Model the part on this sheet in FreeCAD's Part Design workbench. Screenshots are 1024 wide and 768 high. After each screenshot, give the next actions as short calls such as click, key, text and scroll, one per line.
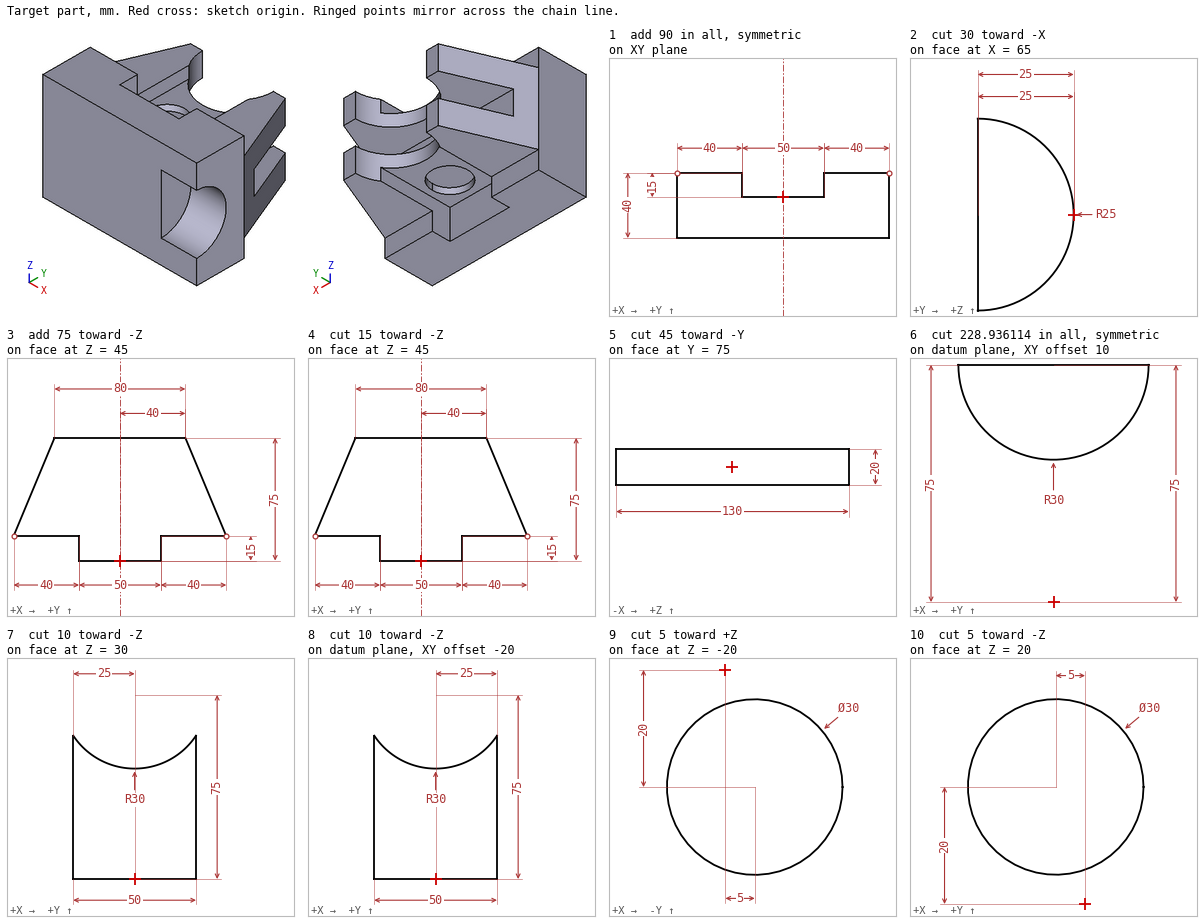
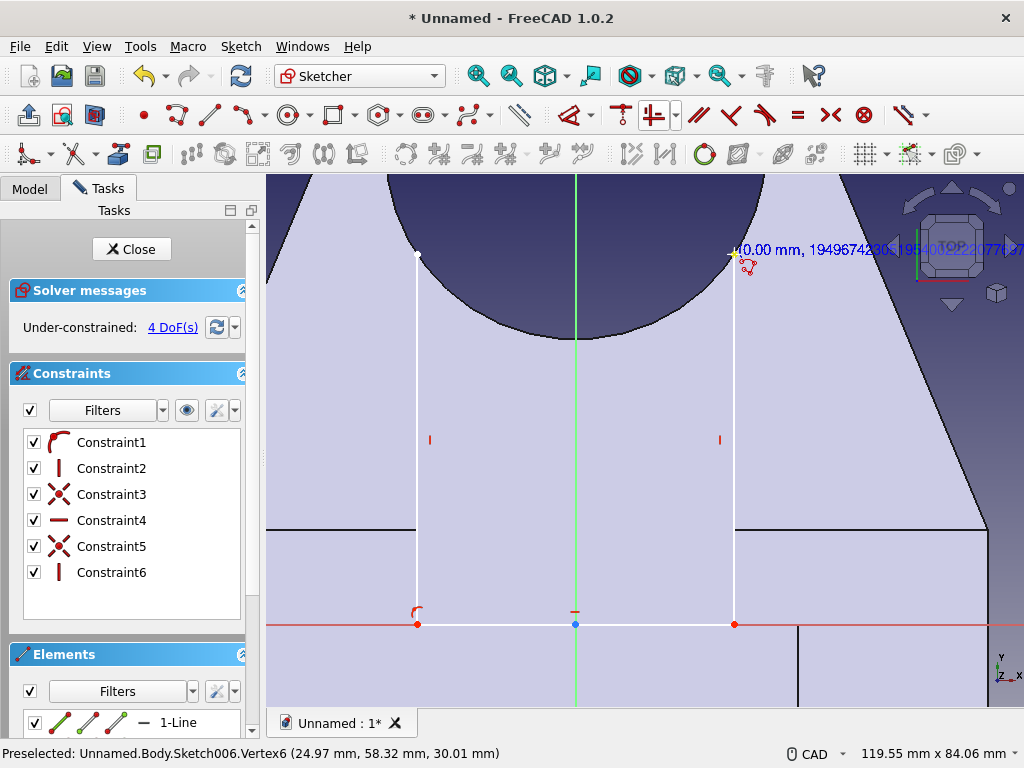
key(g)
key(3)
key(a)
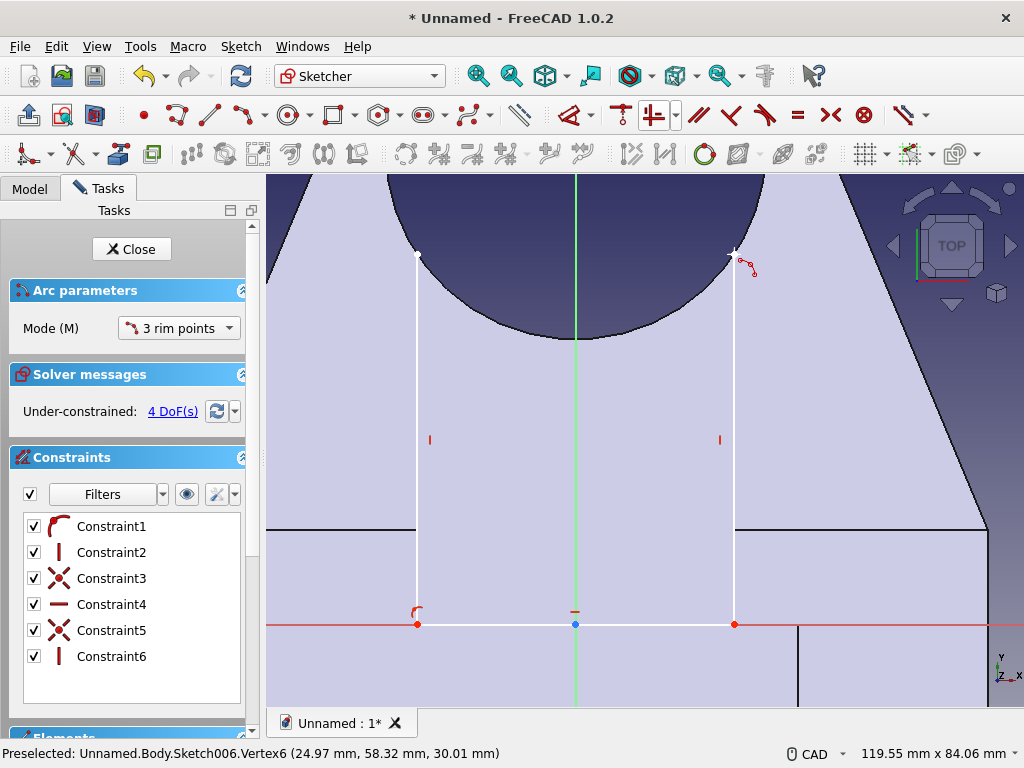
click(734, 255)
click(417, 255)
click(538, 336)
key(Escape)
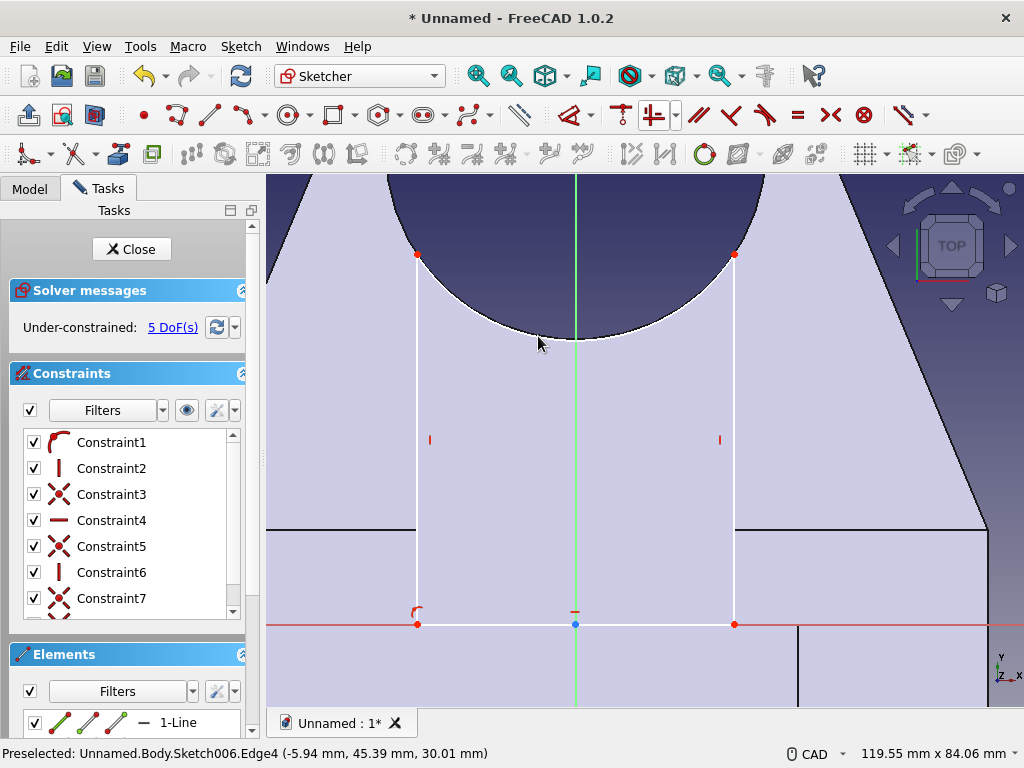
scroll(578, 547, down, 2)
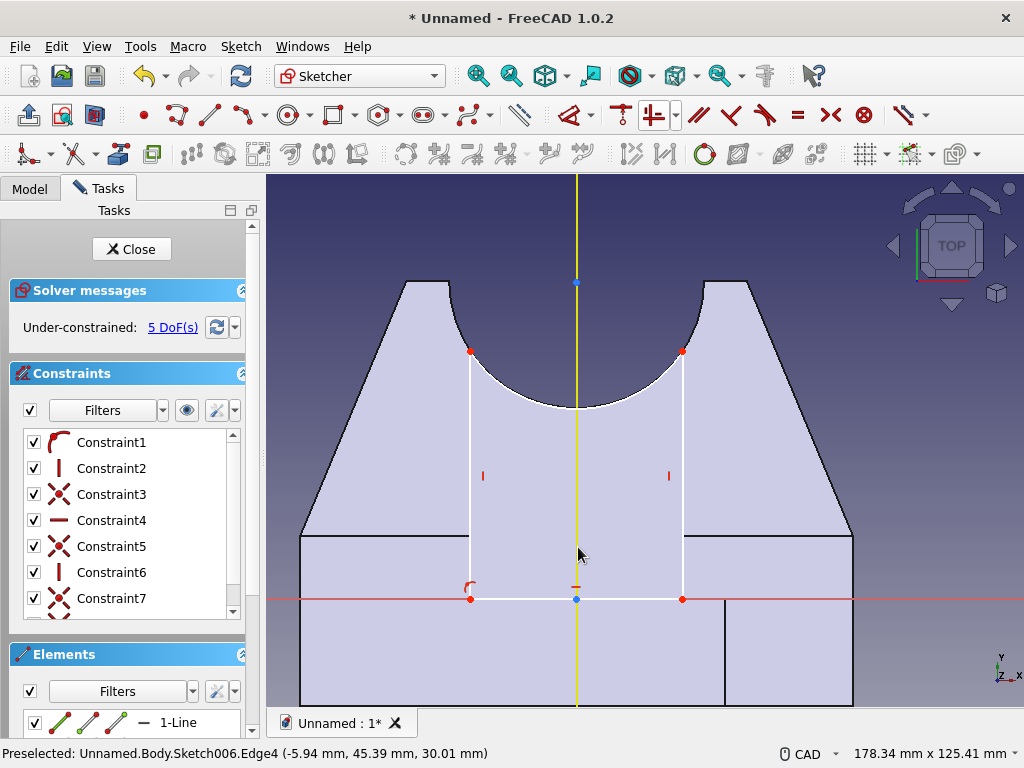
click(576, 282)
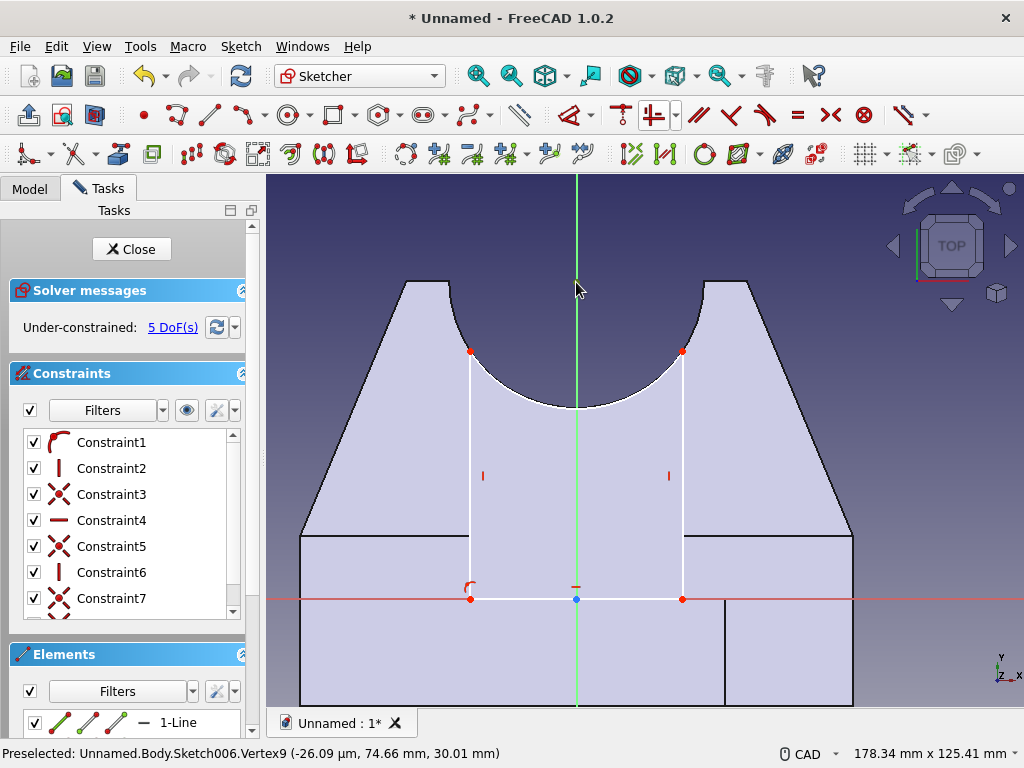
click(577, 645)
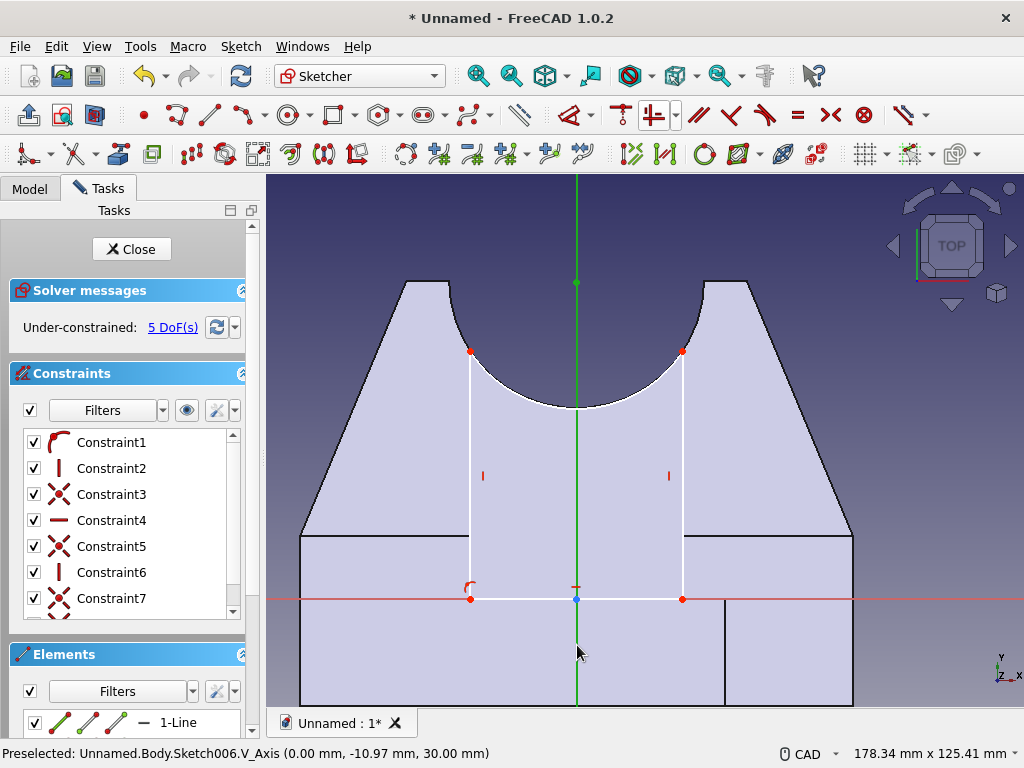
click(621, 116)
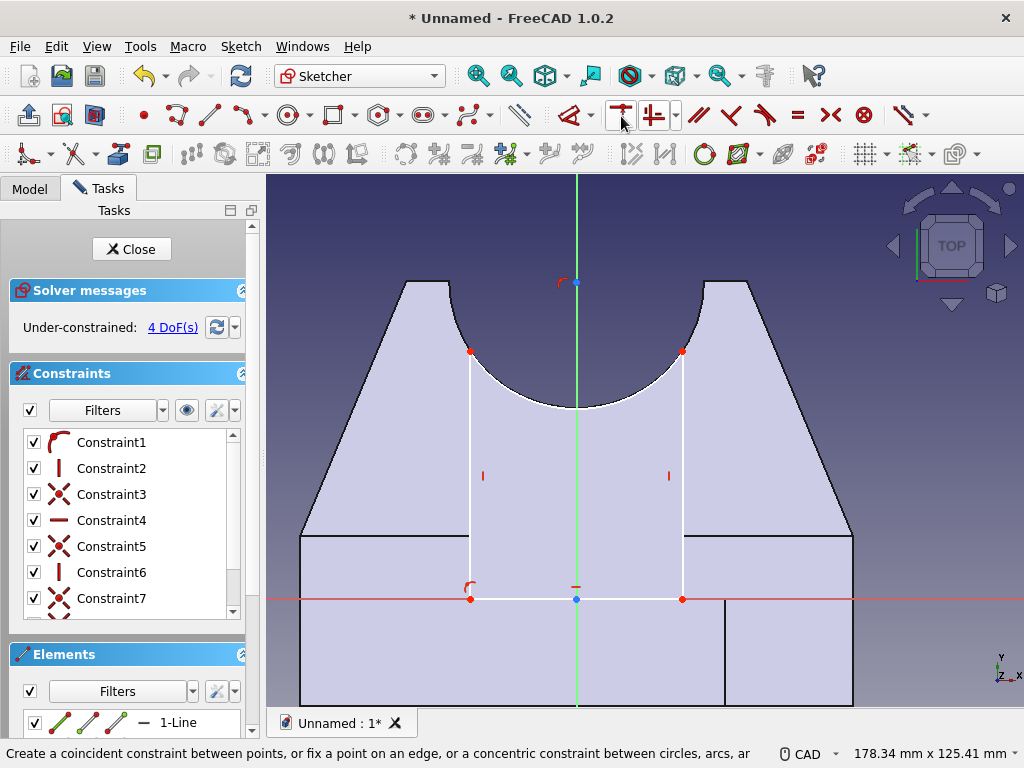
key(d)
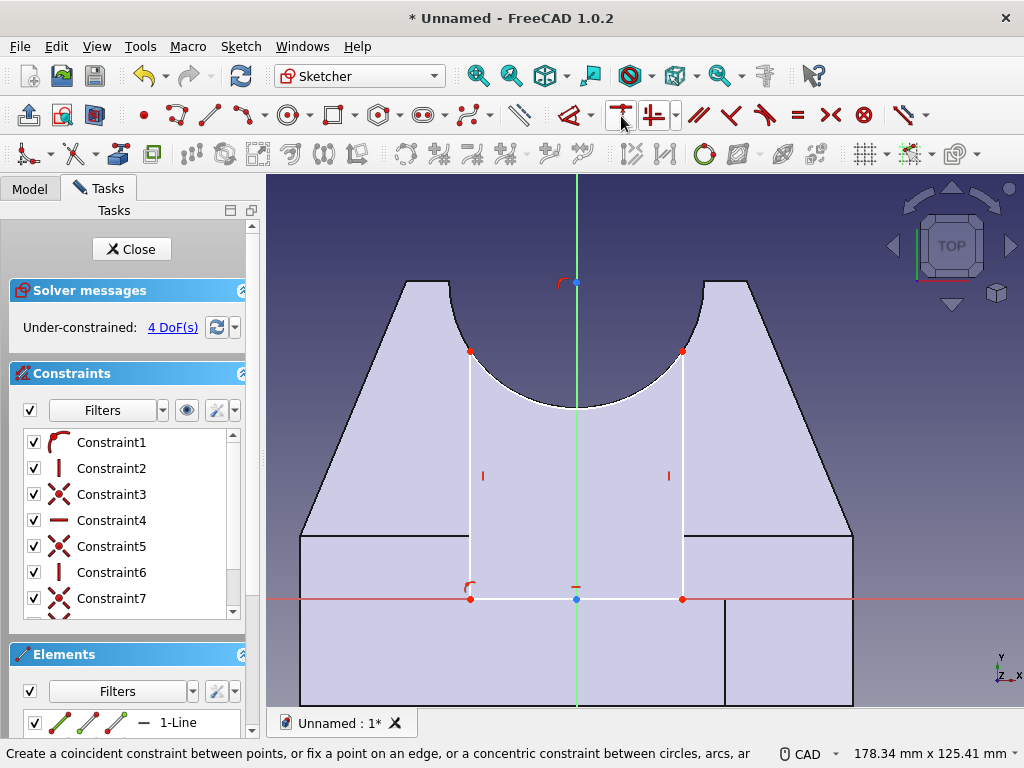
click(527, 399)
click(515, 428)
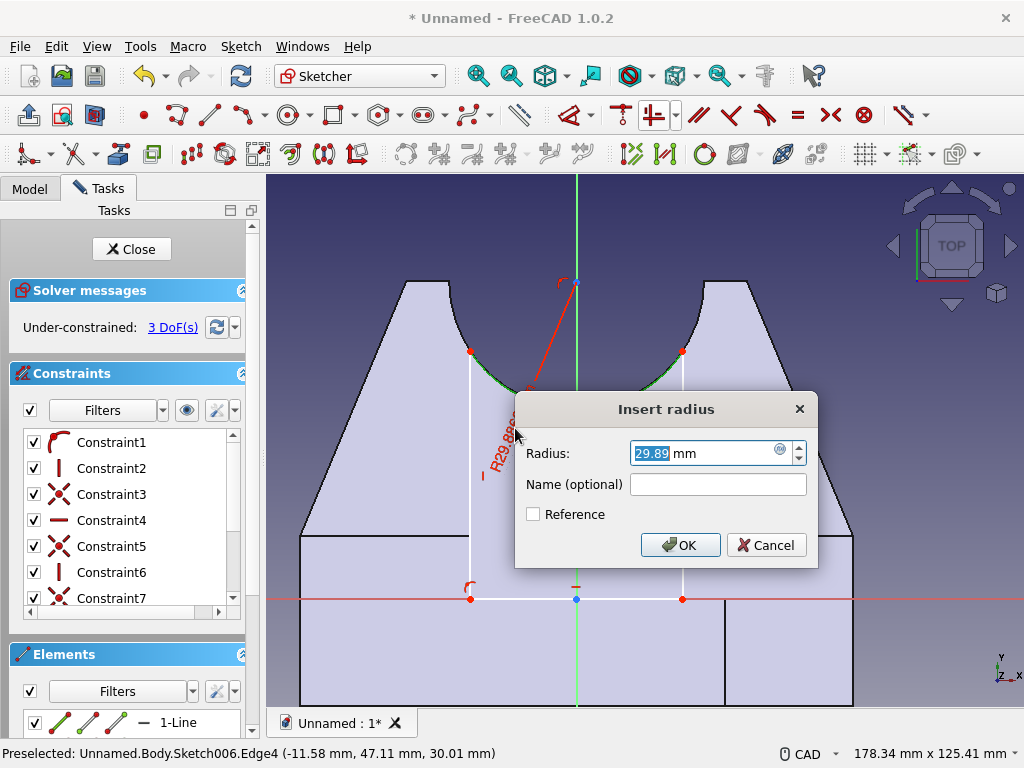
text(30)
key(Return)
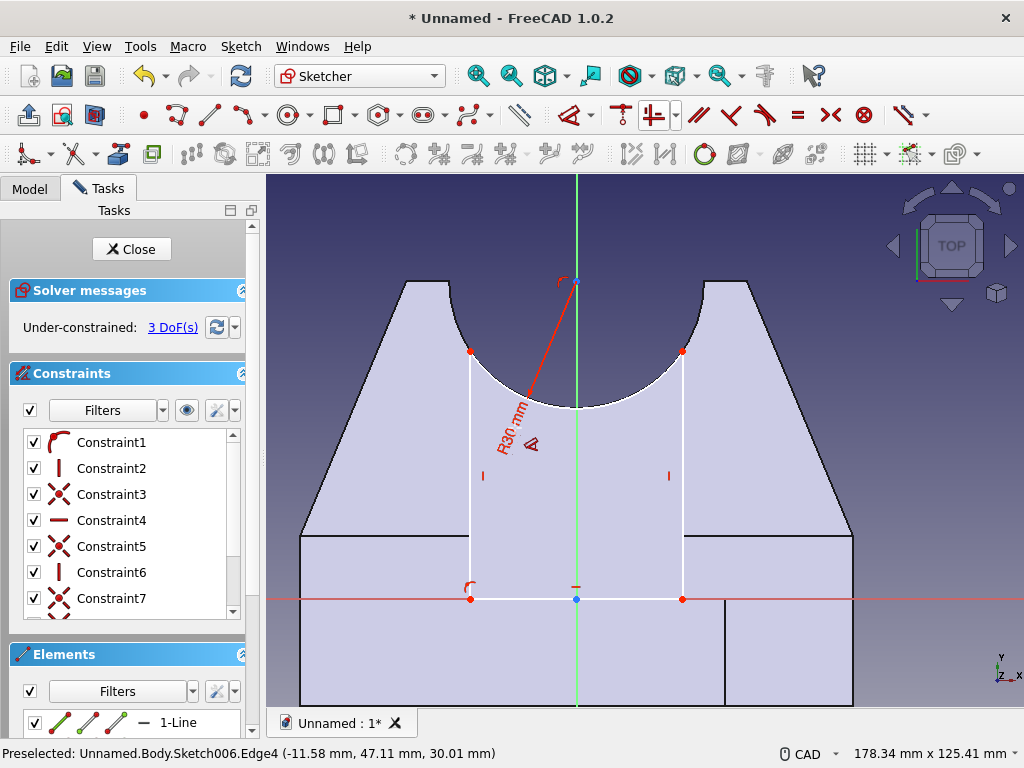
click(534, 599)
click(528, 633)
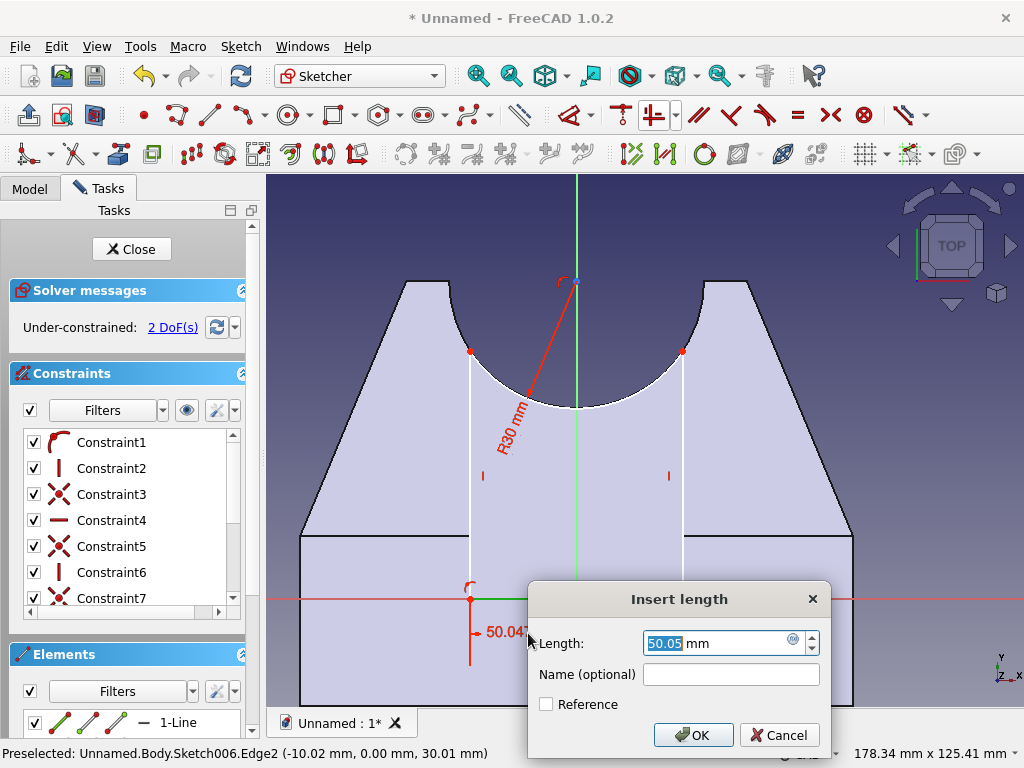
text(50)
key(Return)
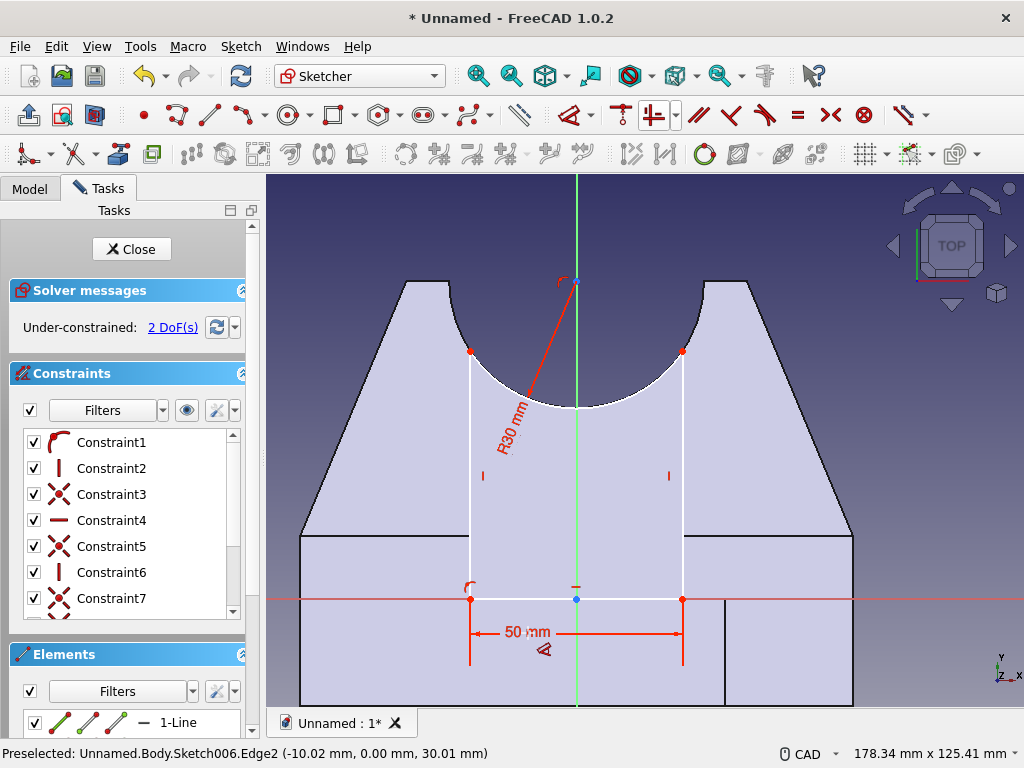
click(470, 351)
click(523, 317)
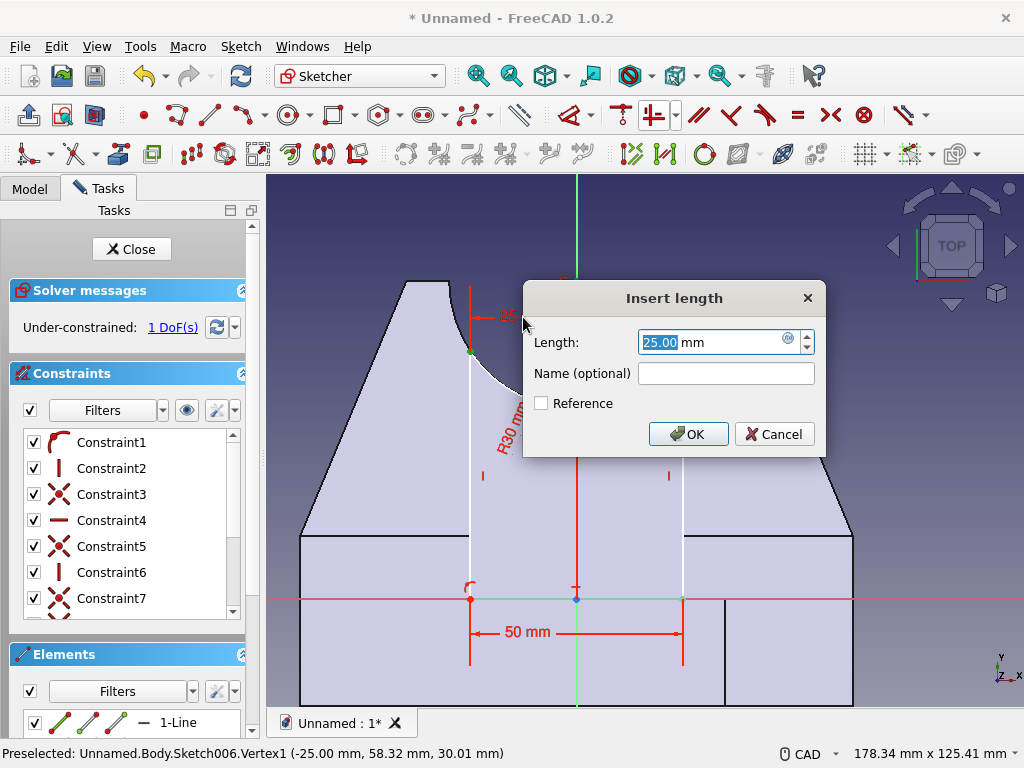
text(25)
key(Return)